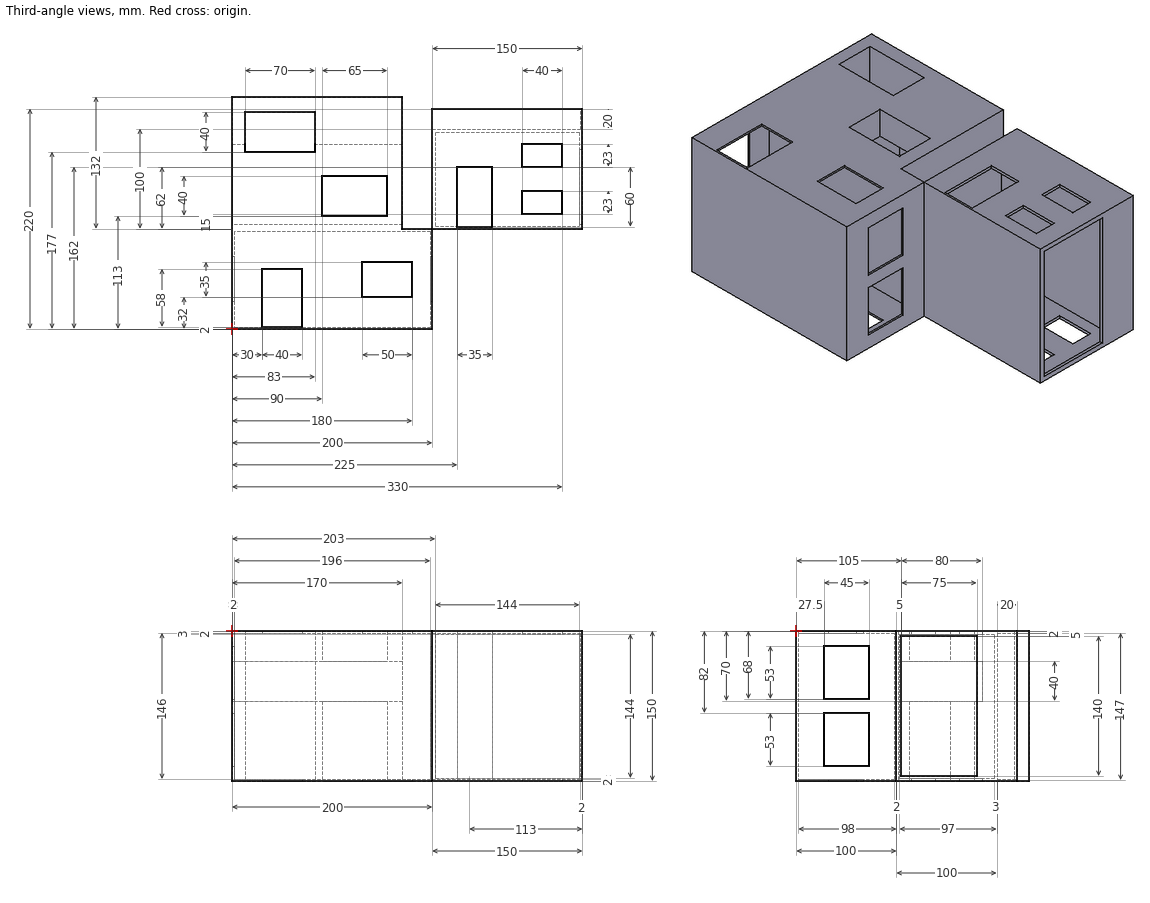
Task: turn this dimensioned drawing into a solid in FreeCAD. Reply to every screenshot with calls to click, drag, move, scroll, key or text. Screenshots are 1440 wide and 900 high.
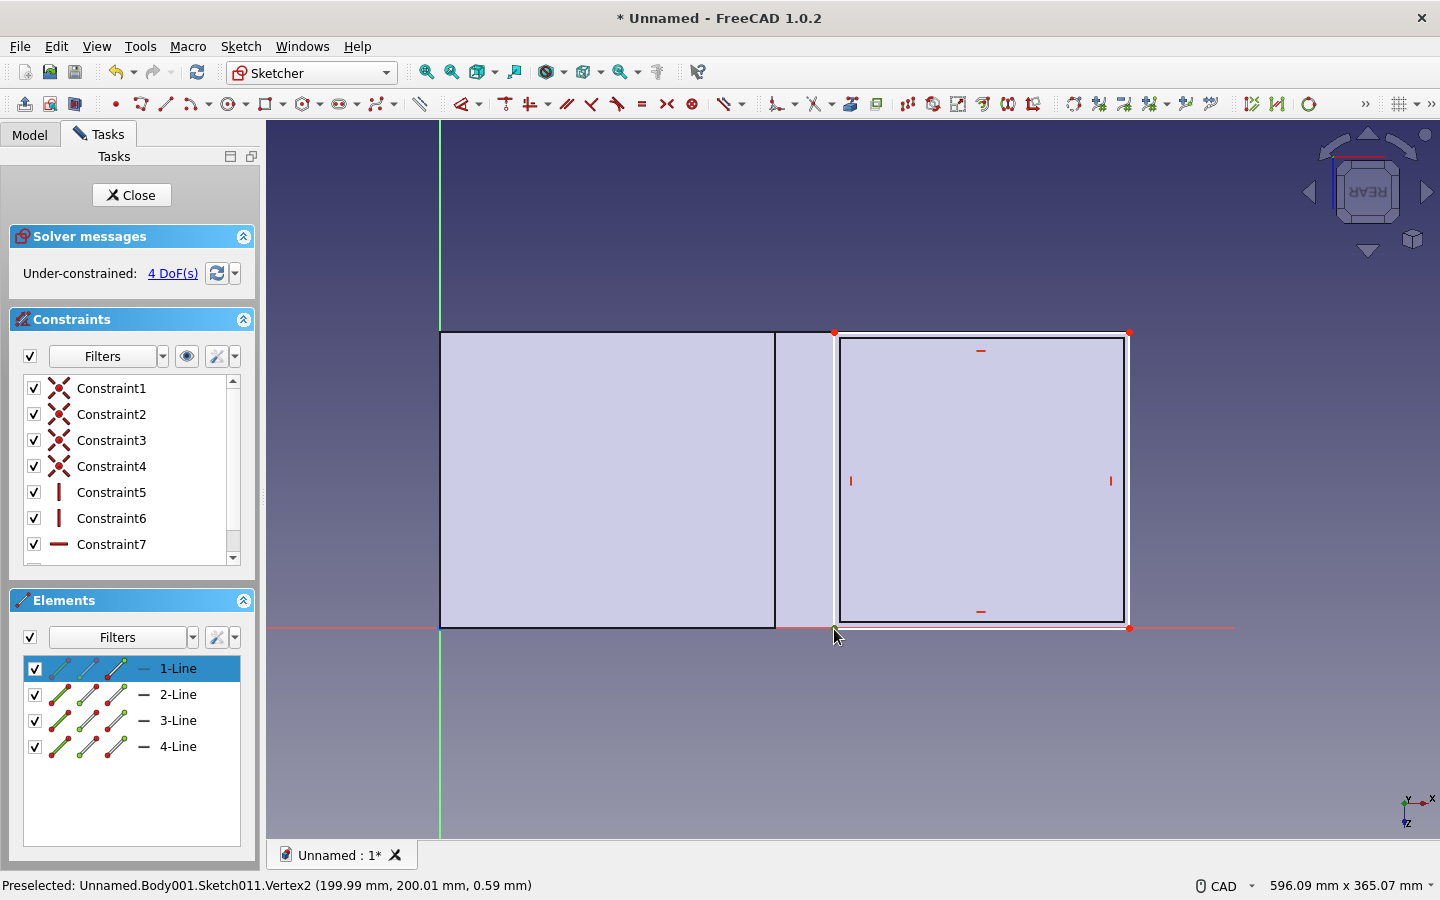
click(364, 628)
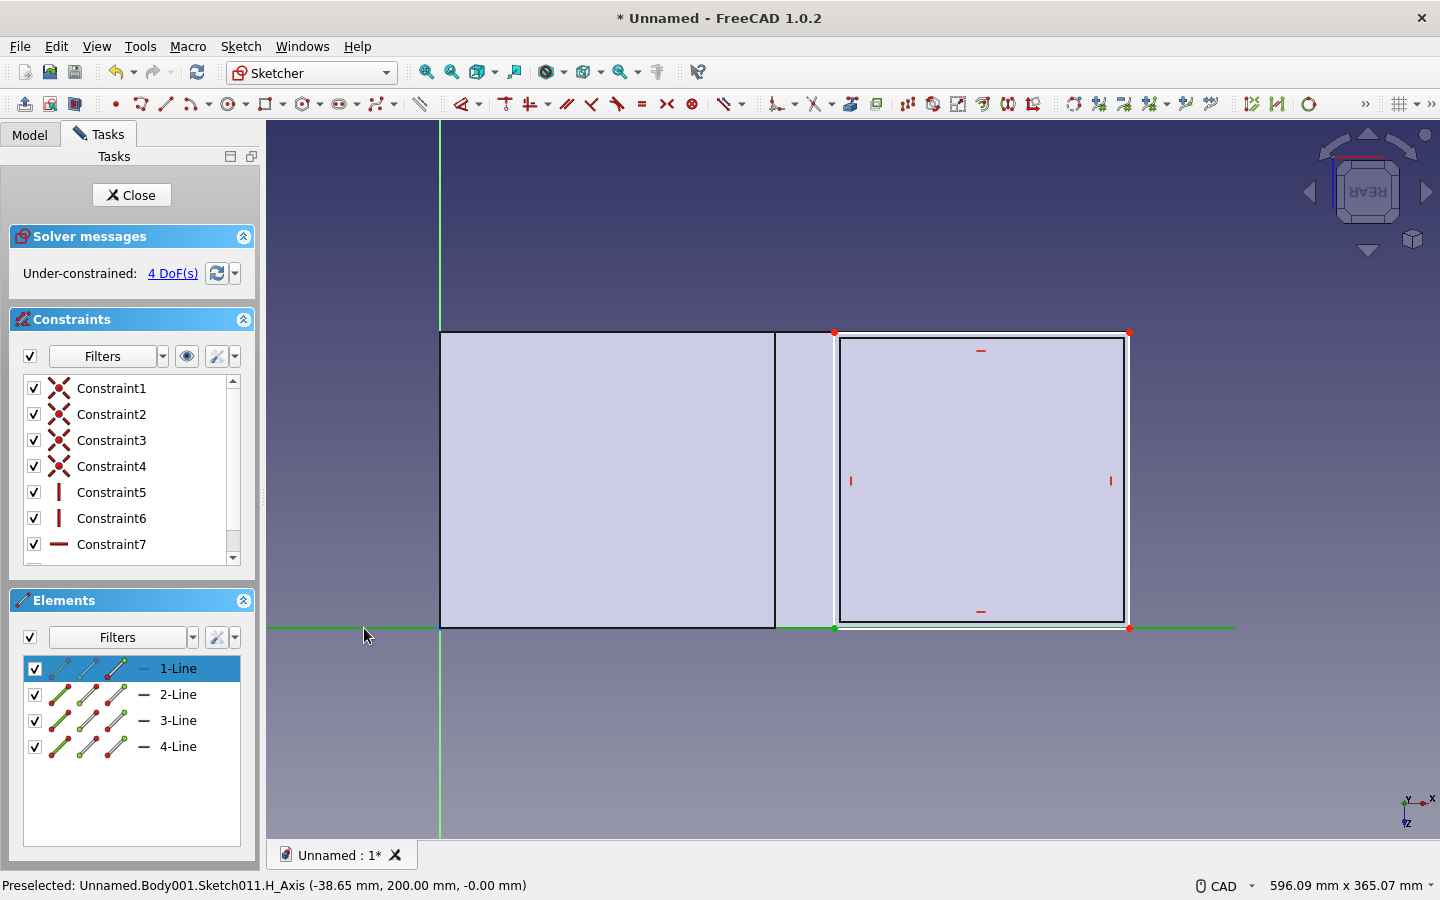
click(505, 104)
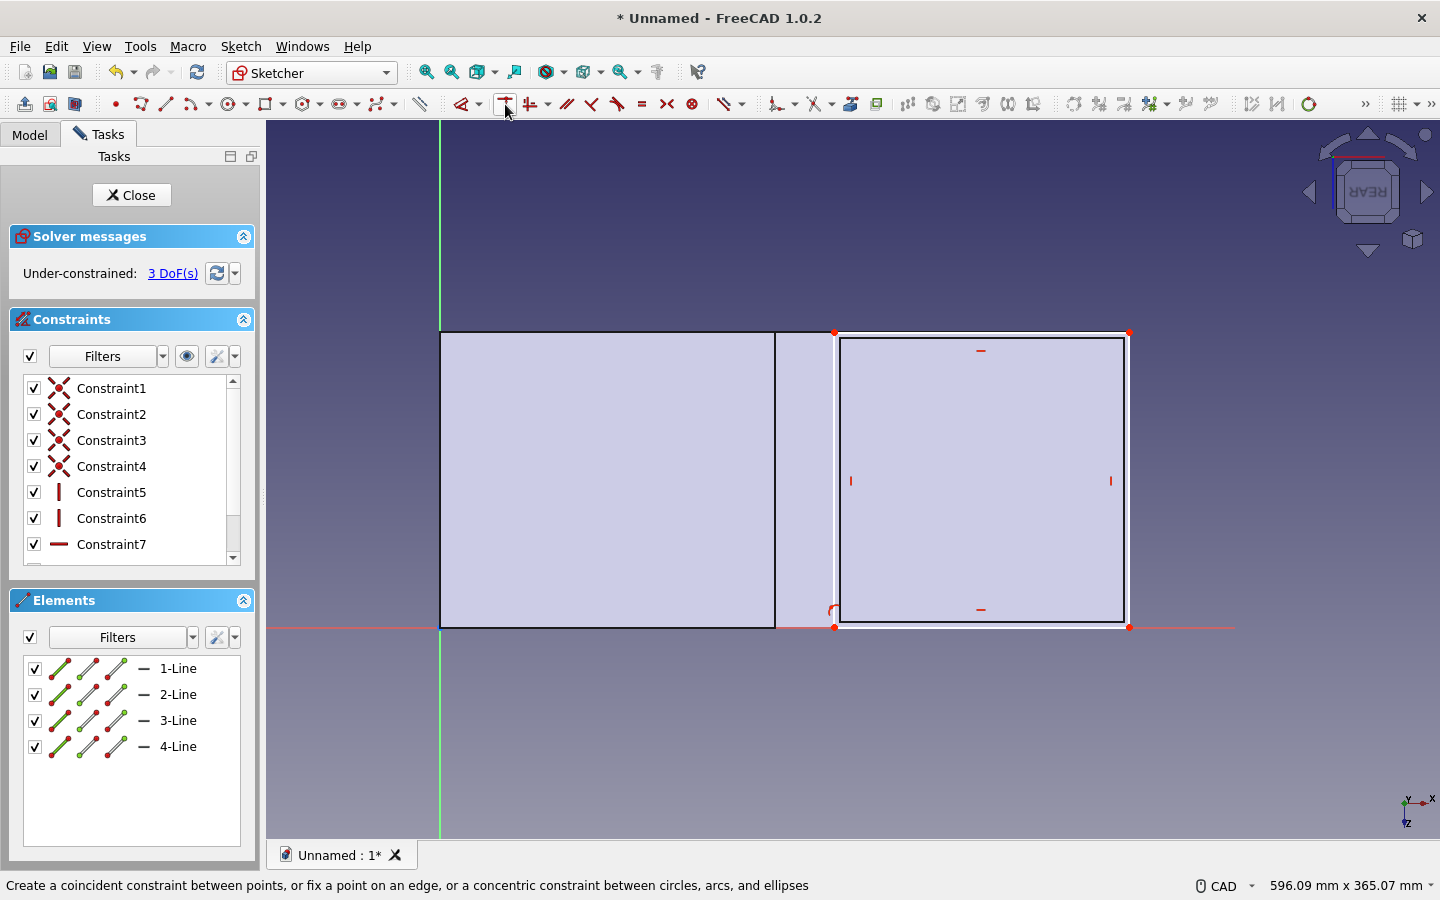
click(460, 104)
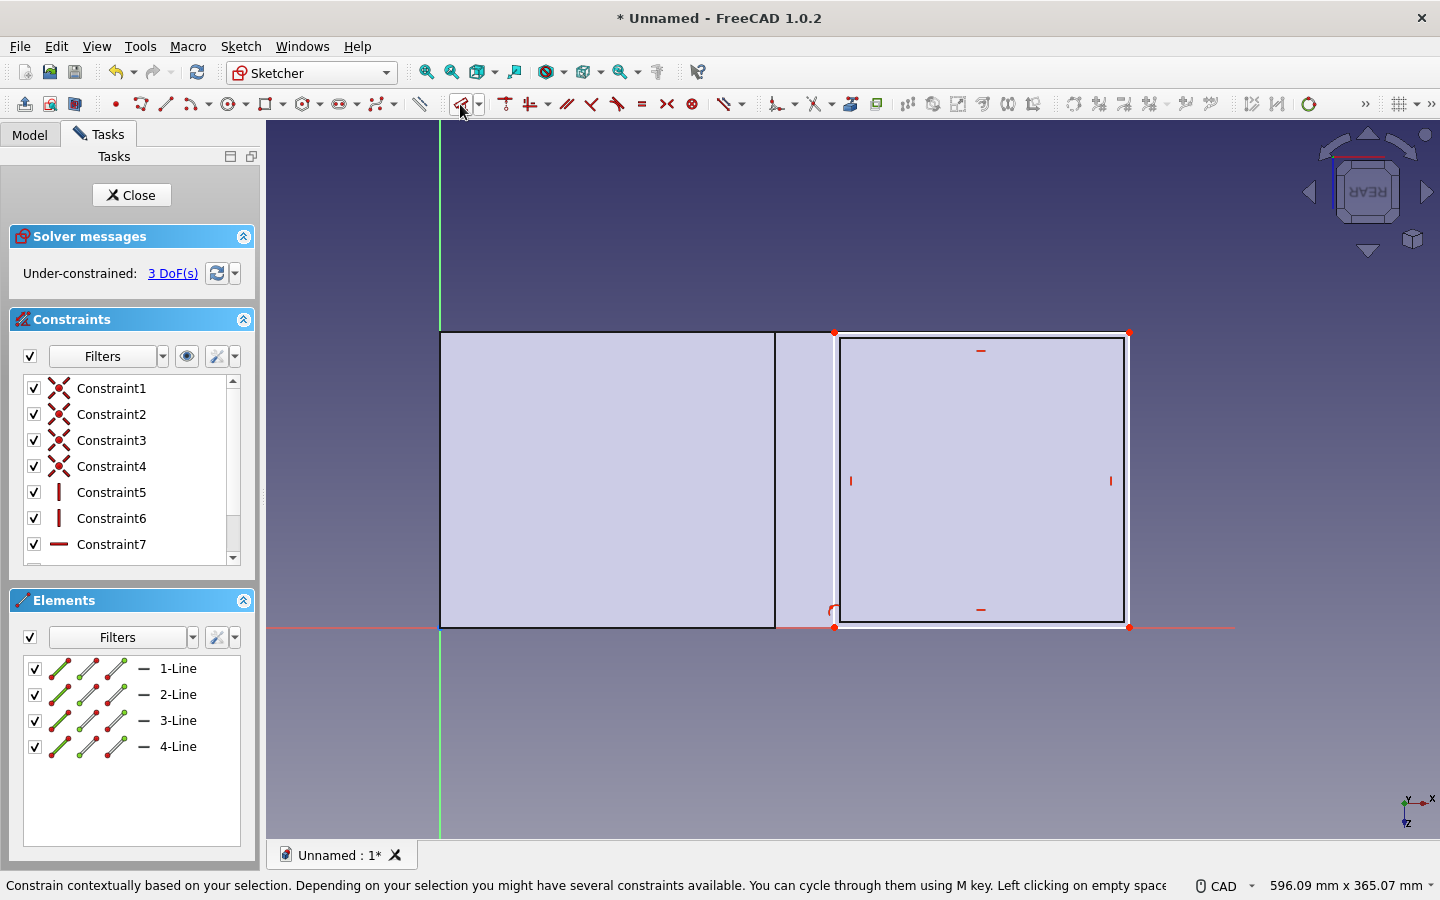
click(834, 421)
click(868, 480)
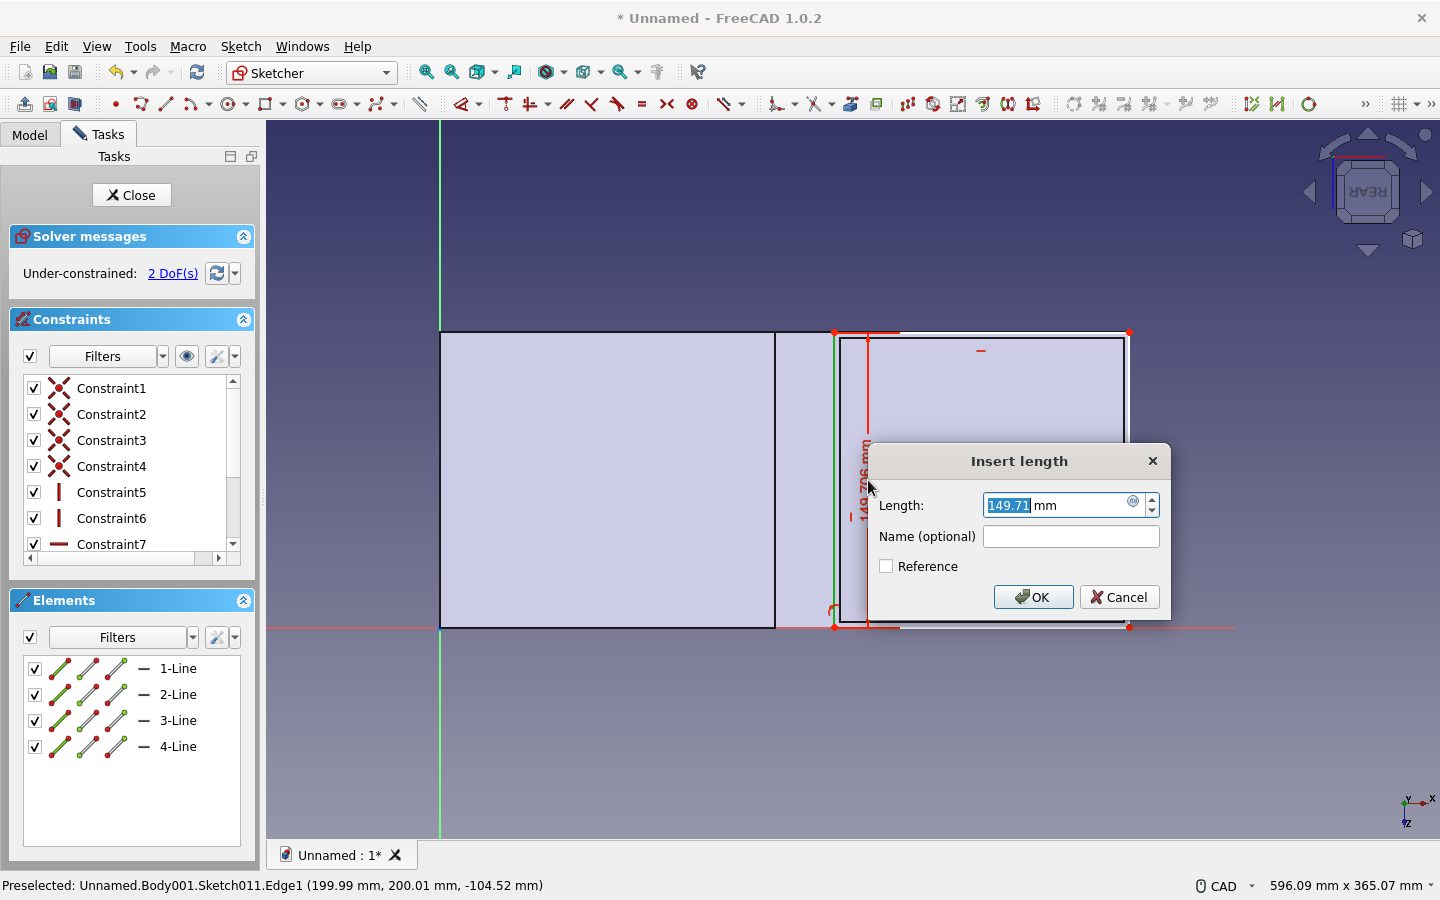
text(150)
key(Return)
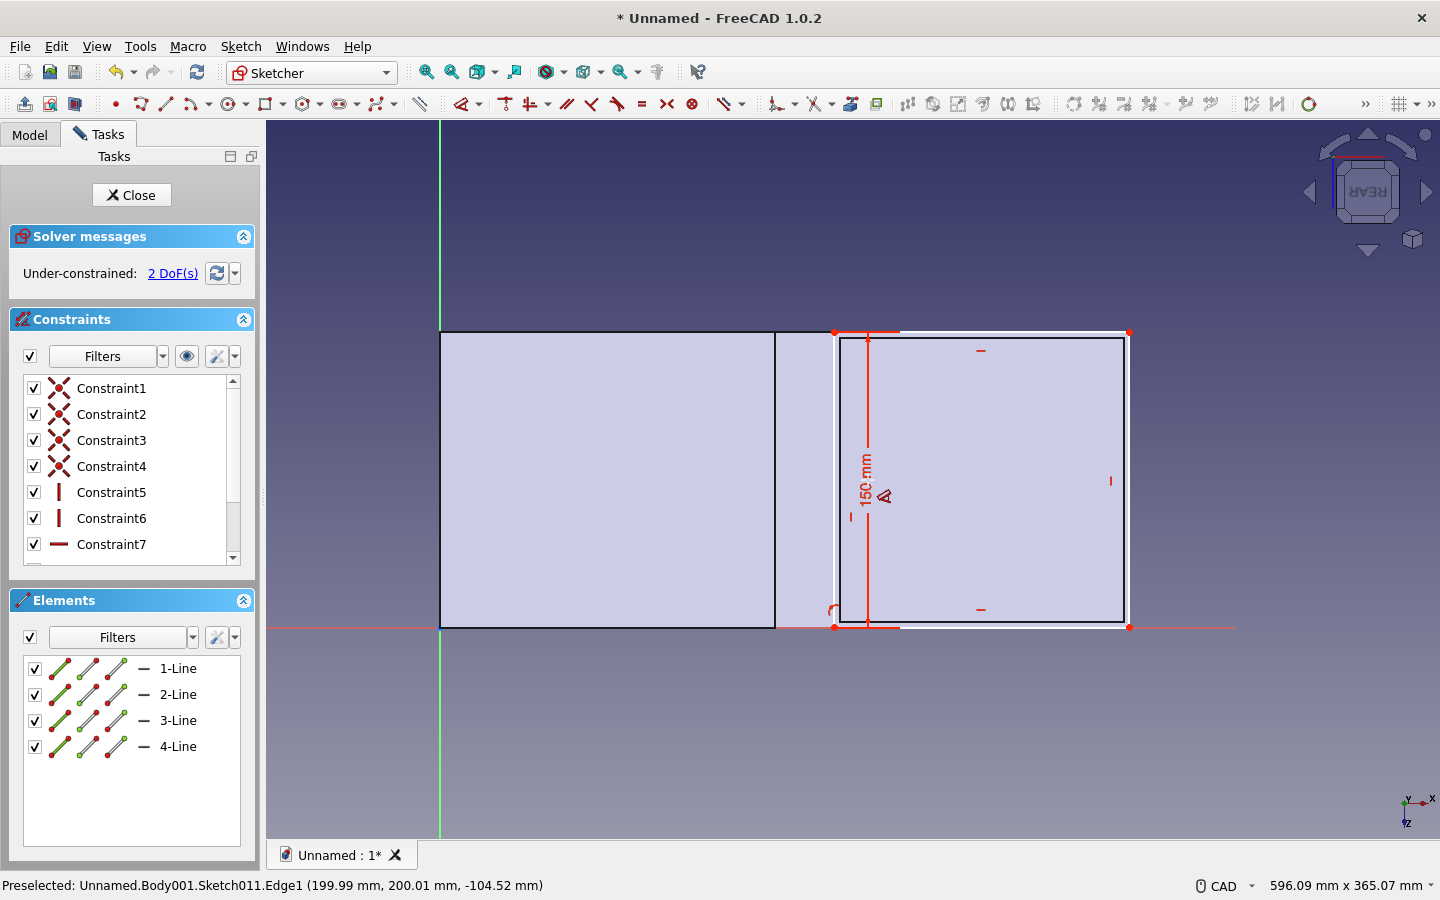
click(923, 628)
click(982, 662)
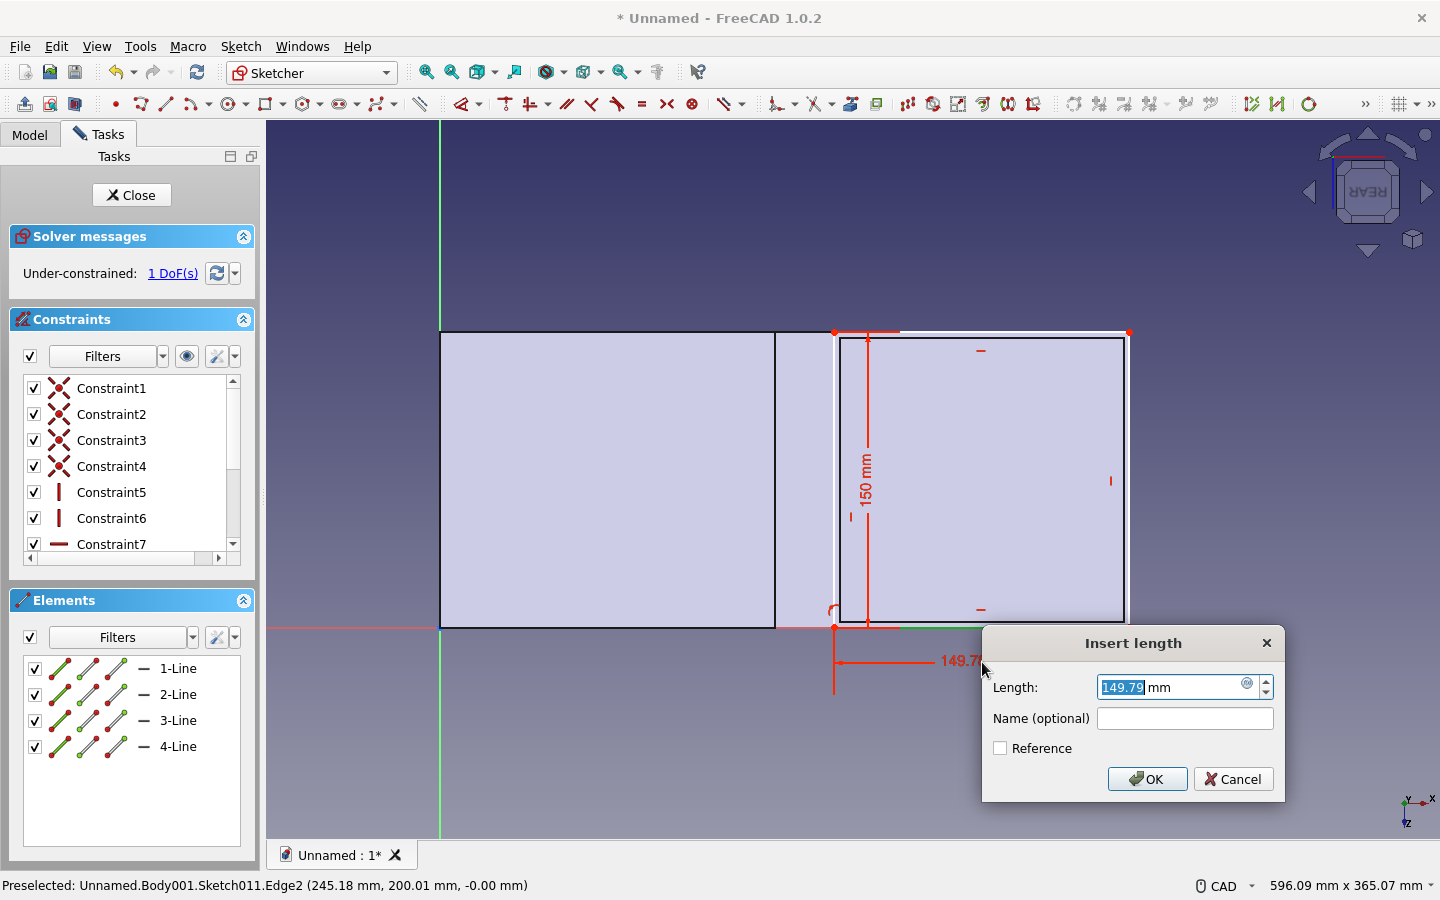
text(150)
key(Return)